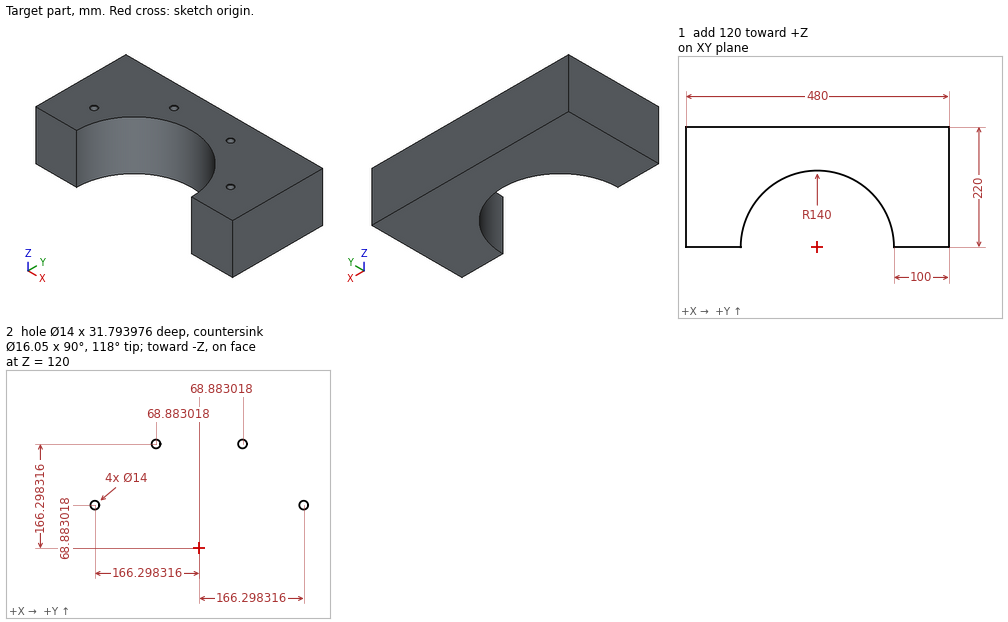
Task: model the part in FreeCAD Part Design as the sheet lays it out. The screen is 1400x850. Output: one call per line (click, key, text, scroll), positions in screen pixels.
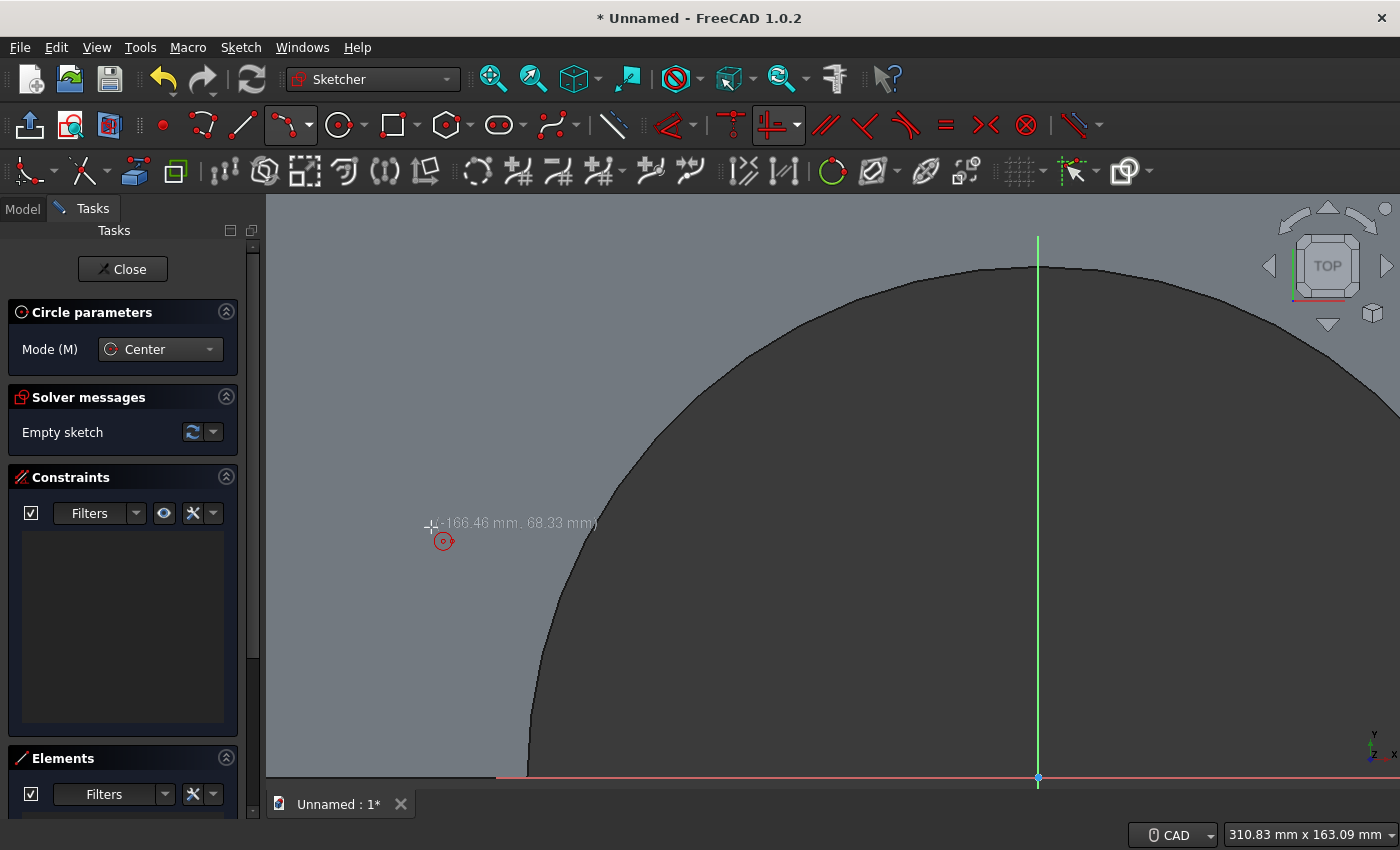
click(431, 526)
click(450, 508)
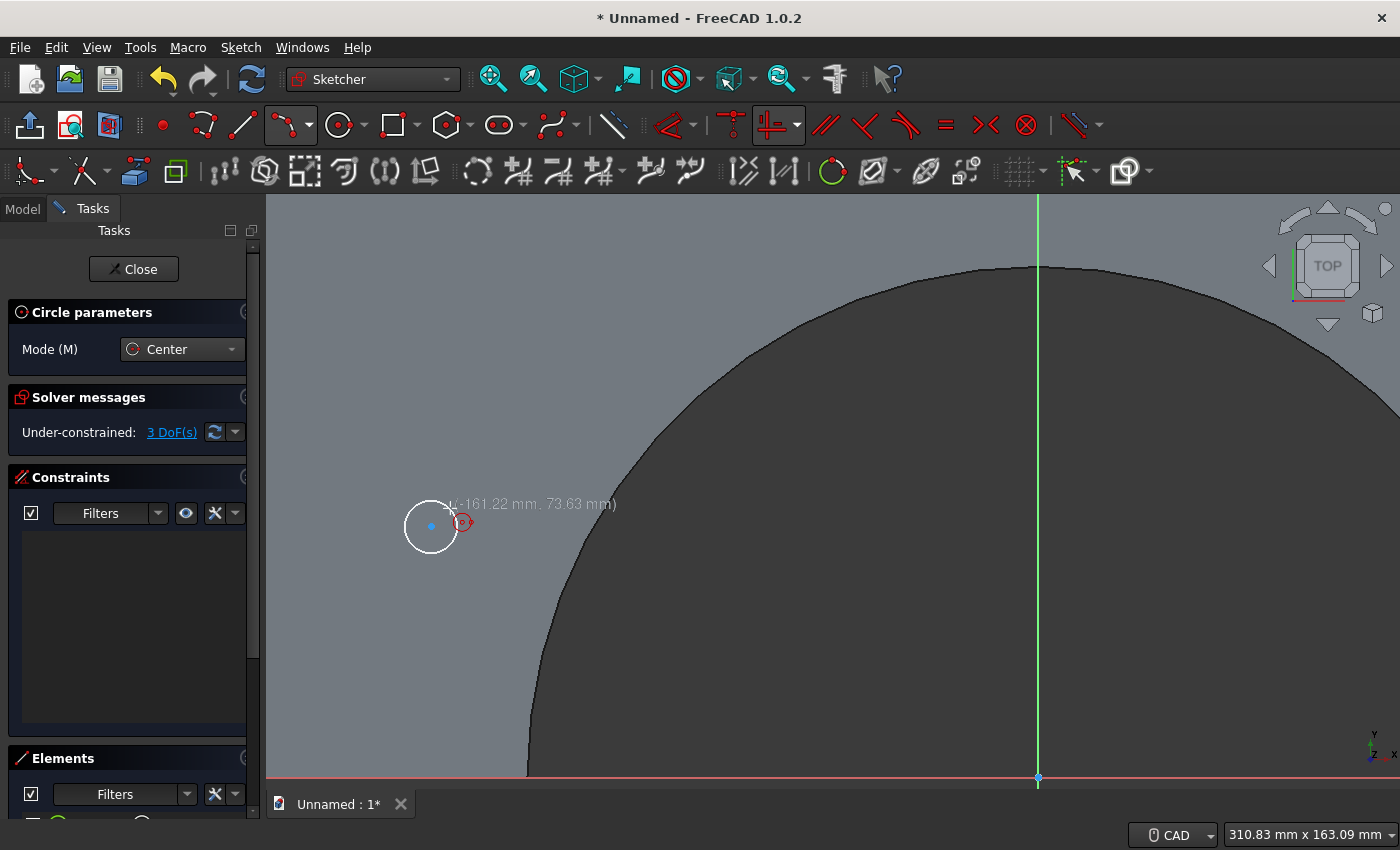
scroll(432, 528, down, 3)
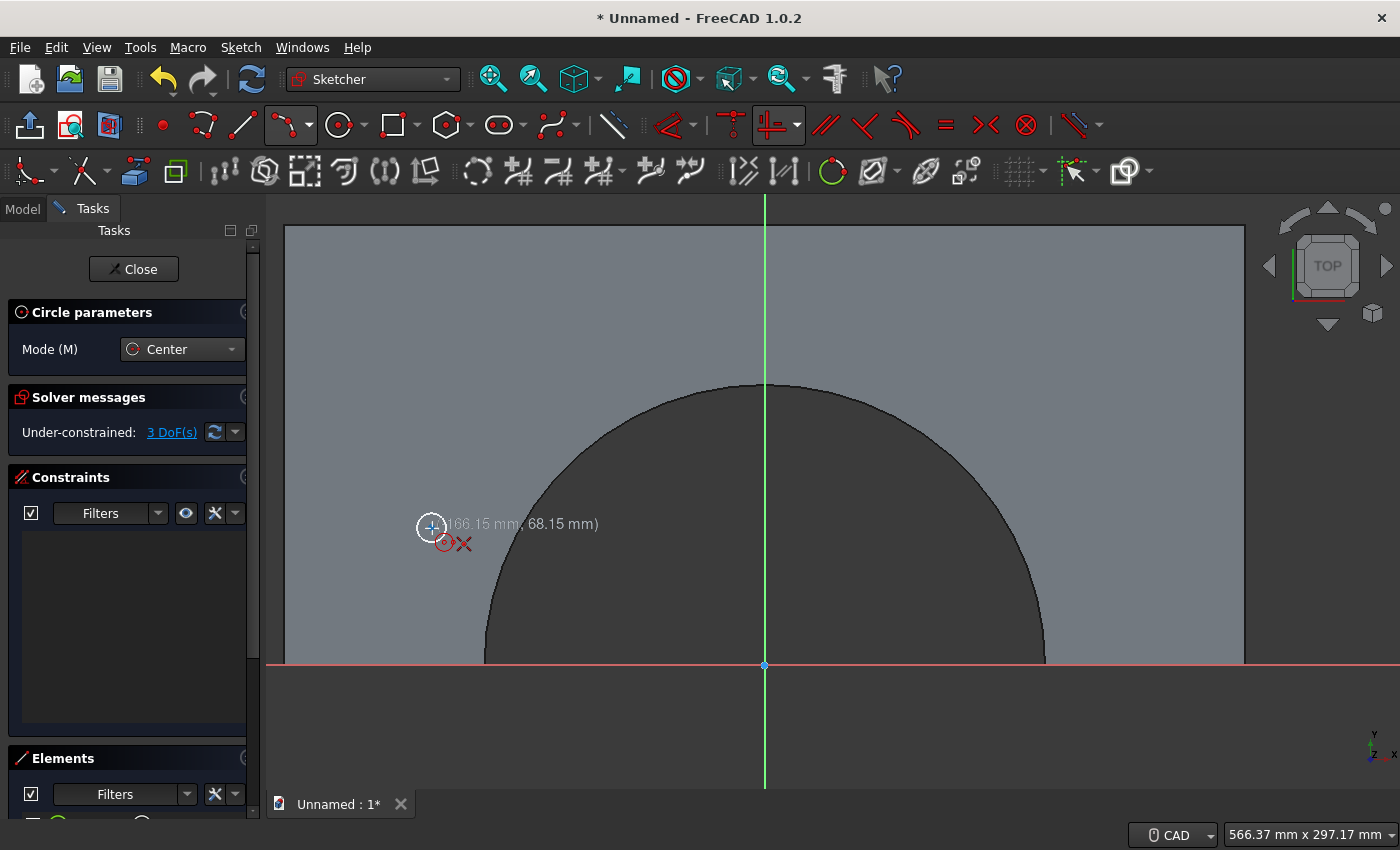
scroll(627, 332, up, 3)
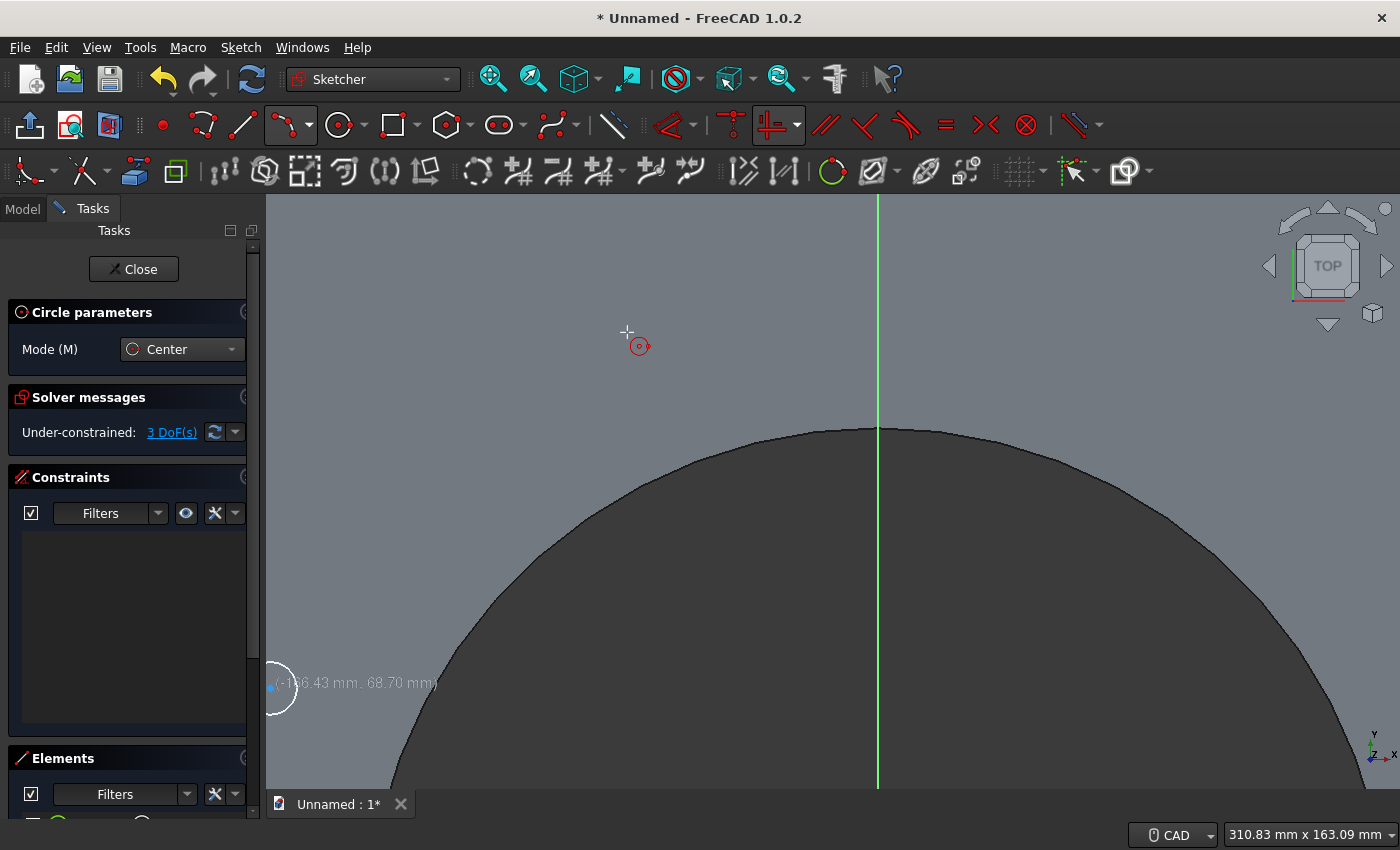
click(626, 332)
click(644, 314)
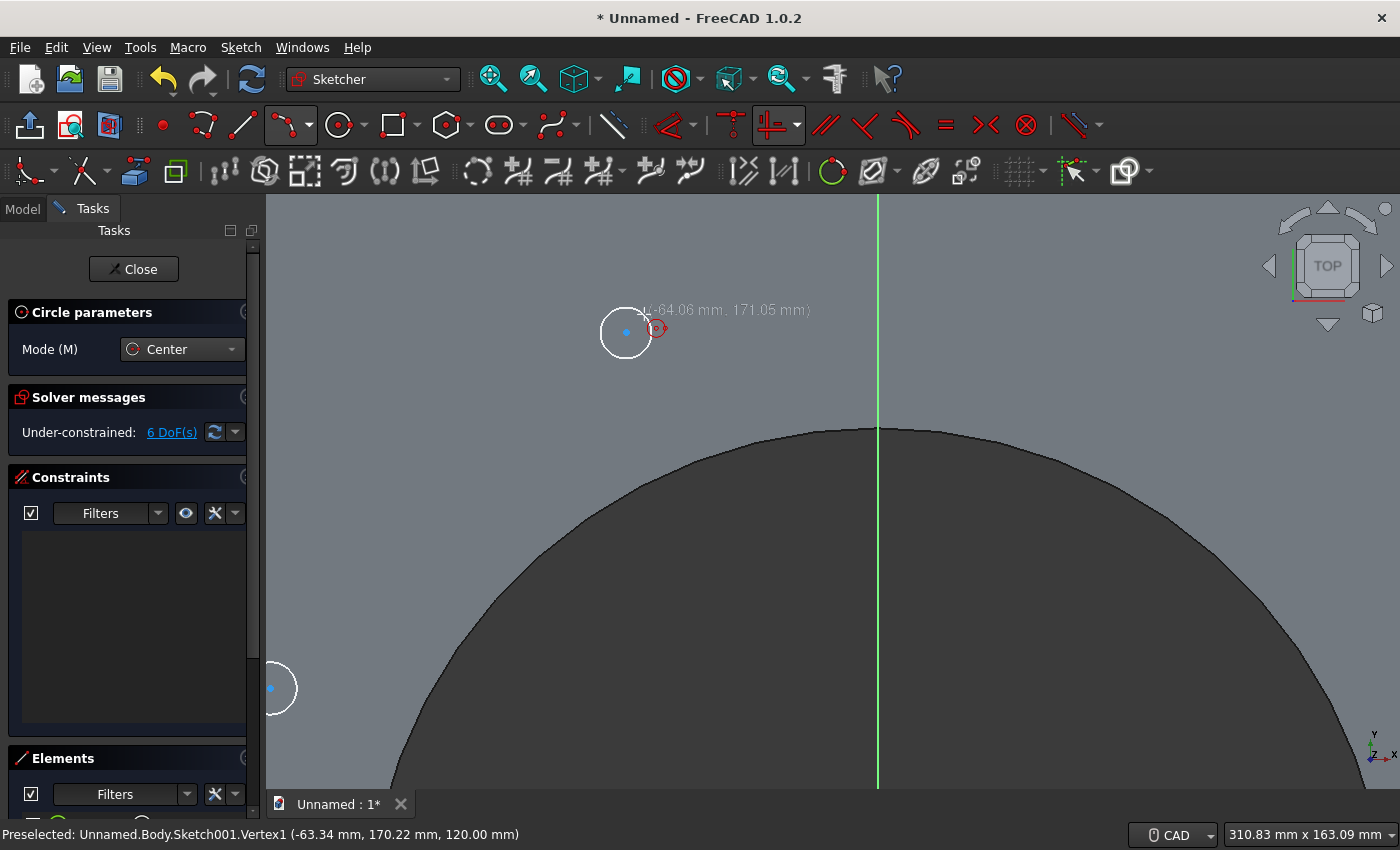
click(1129, 332)
click(1147, 314)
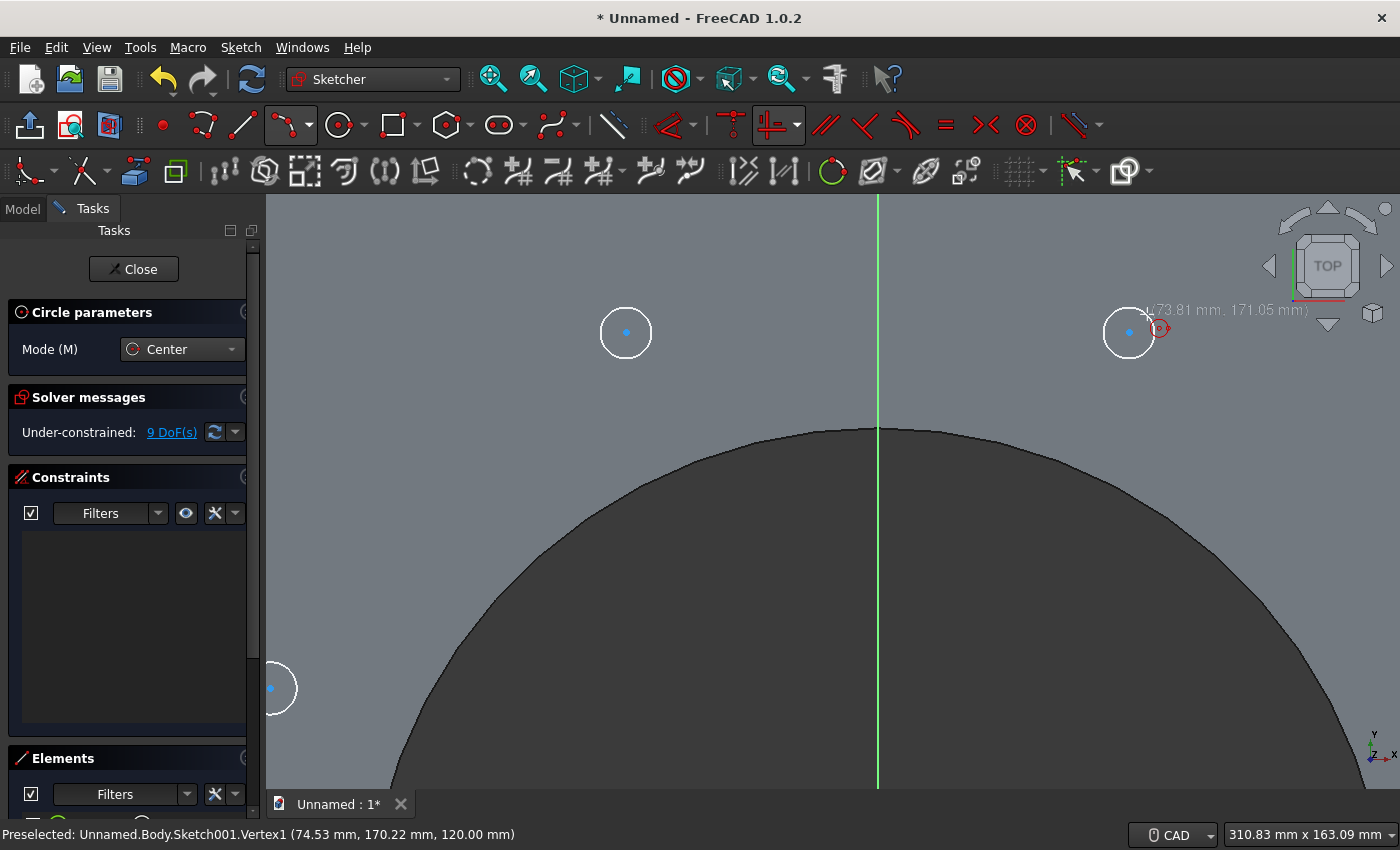
scroll(627, 332, down, 3)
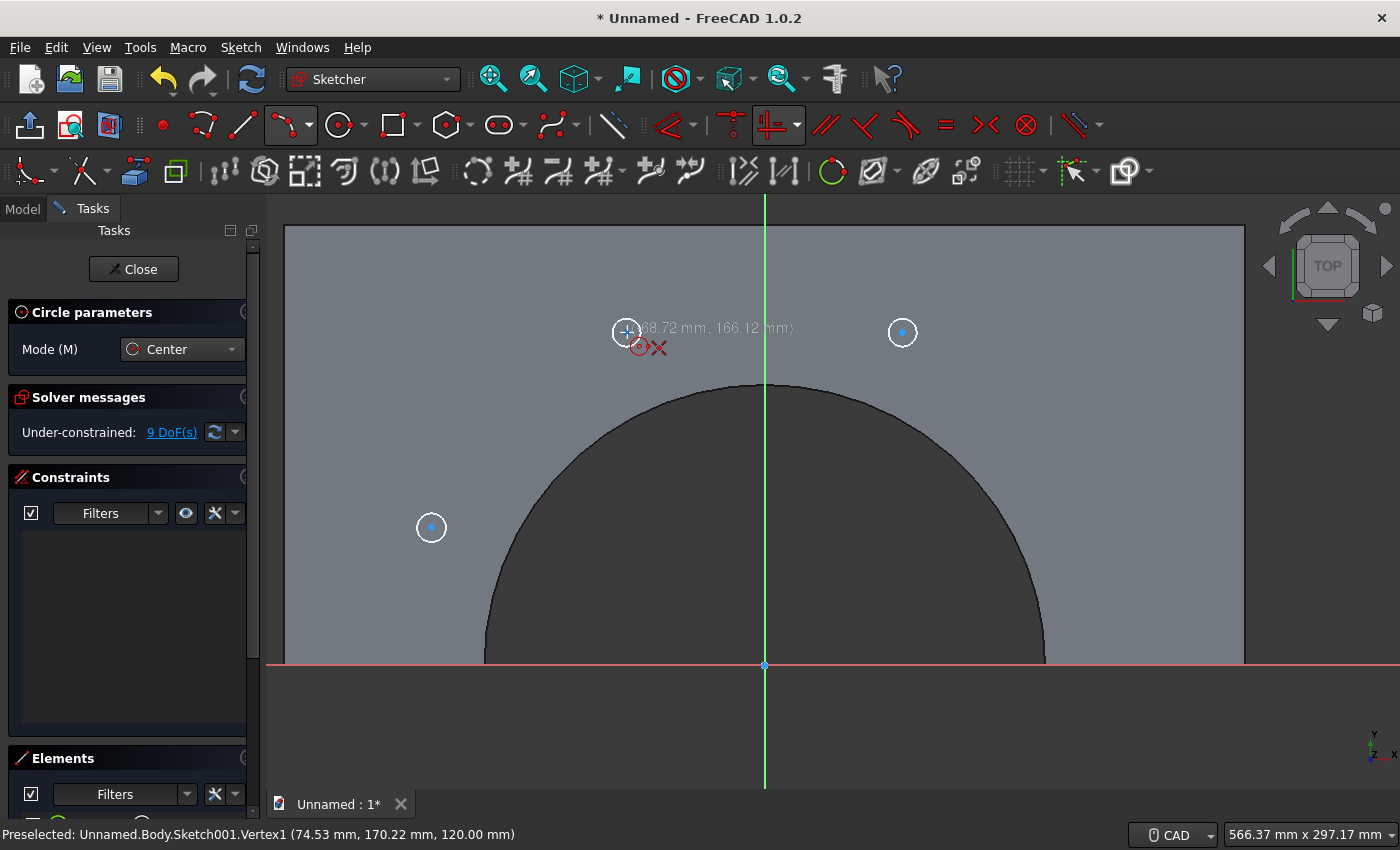
scroll(1098, 527, up, 3)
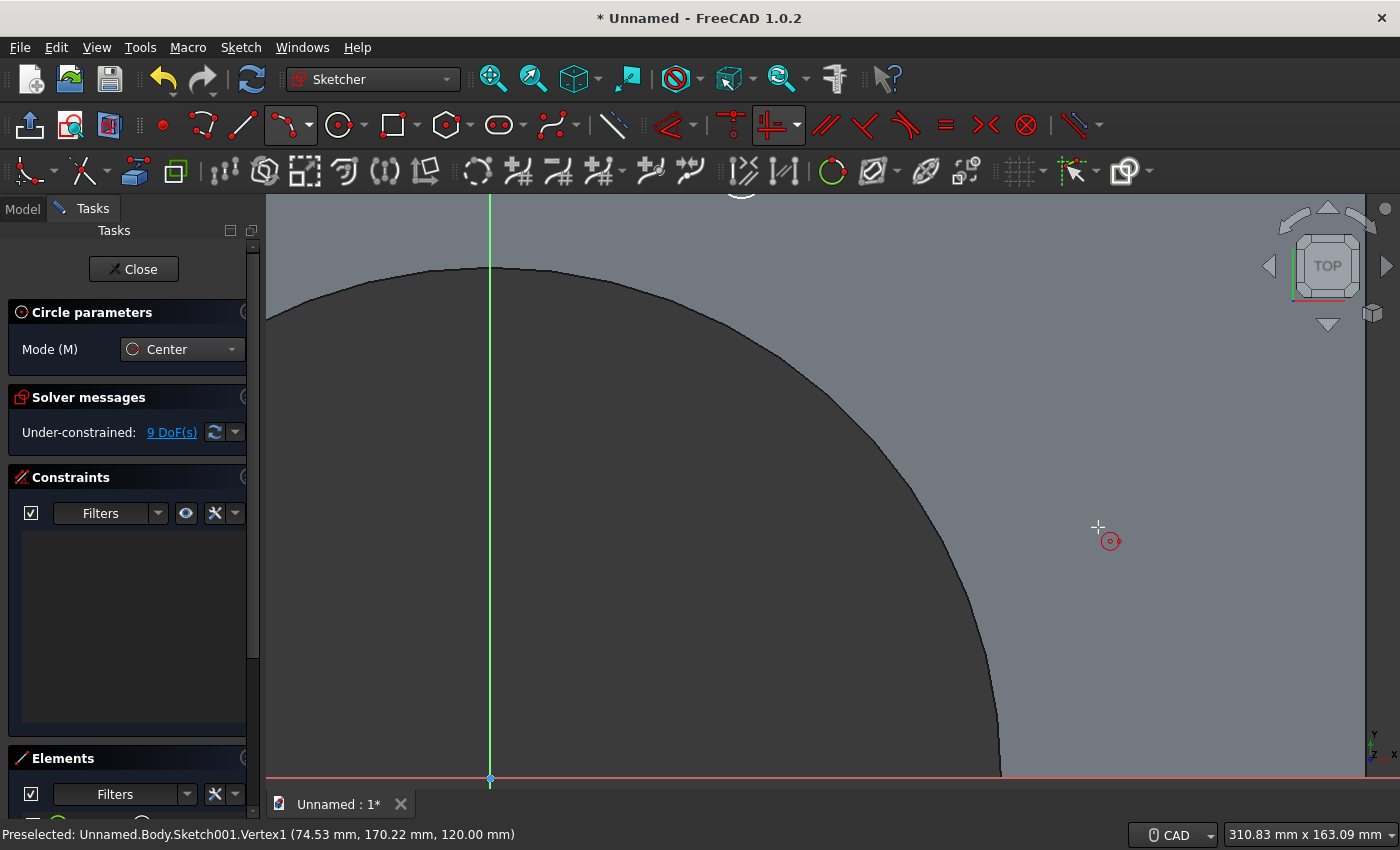
click(1097, 527)
click(1115, 509)
key(Escape)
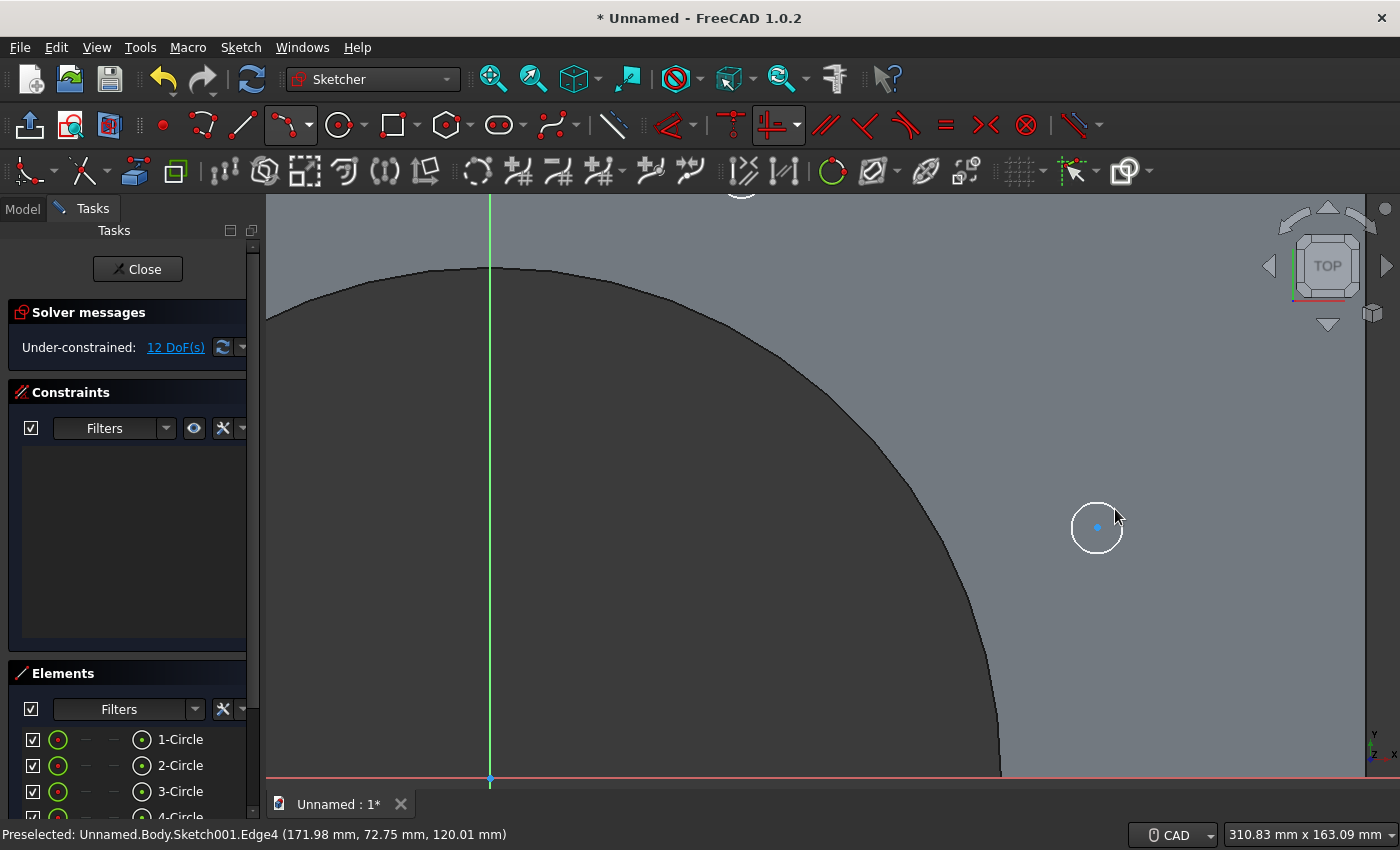
scroll(1098, 527, down, 3)